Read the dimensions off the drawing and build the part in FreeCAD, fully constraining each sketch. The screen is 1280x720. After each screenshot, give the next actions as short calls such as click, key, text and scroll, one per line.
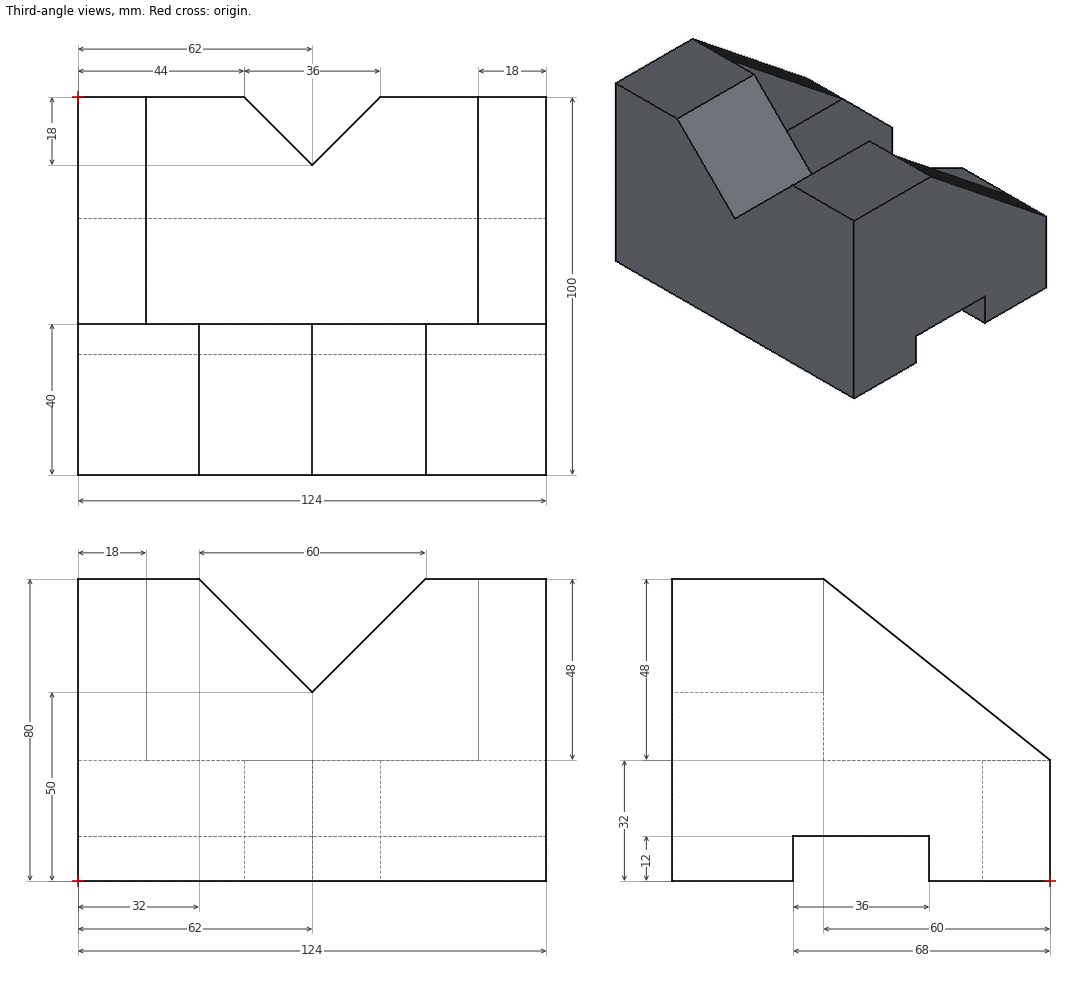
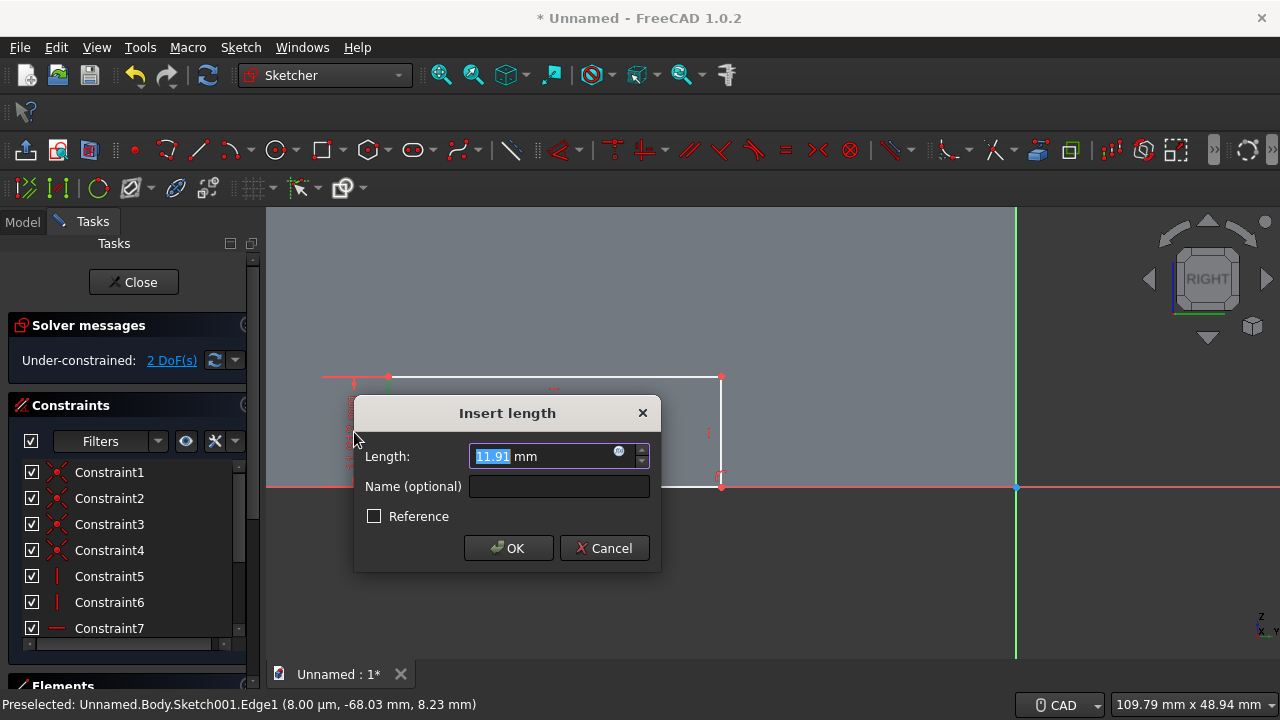
text(12)
key(Return)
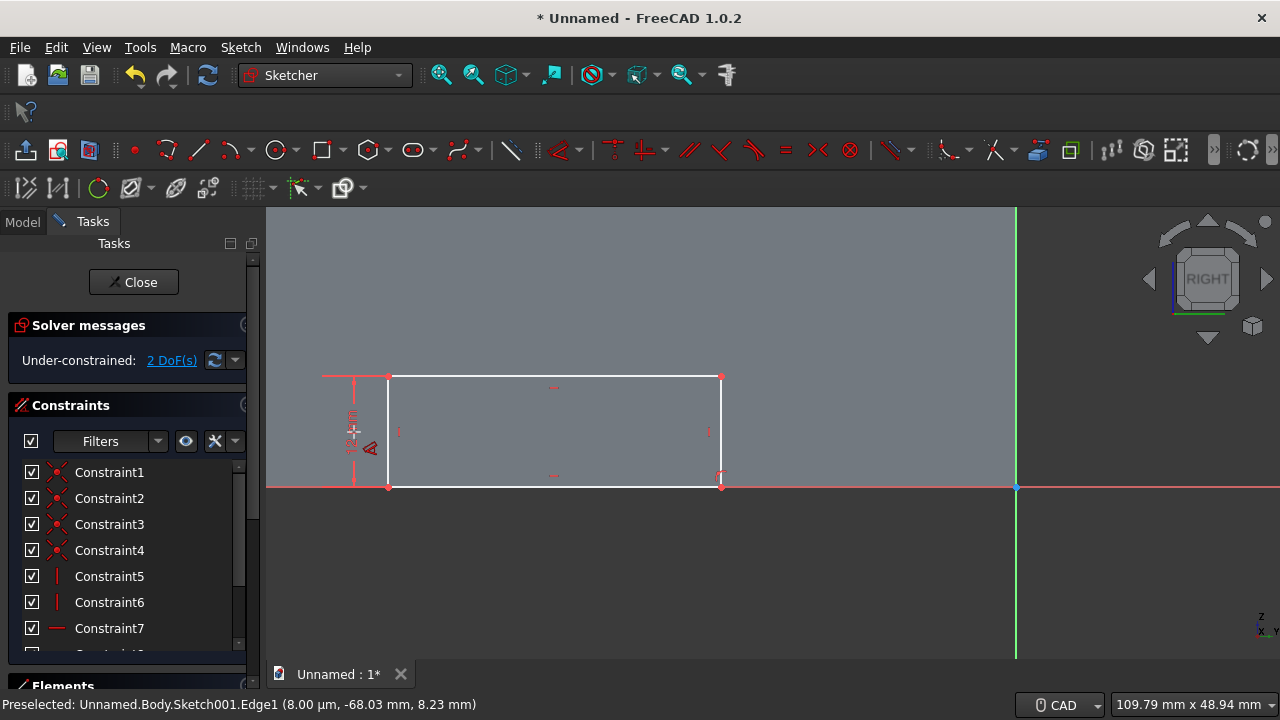
click(488, 487)
click(554, 521)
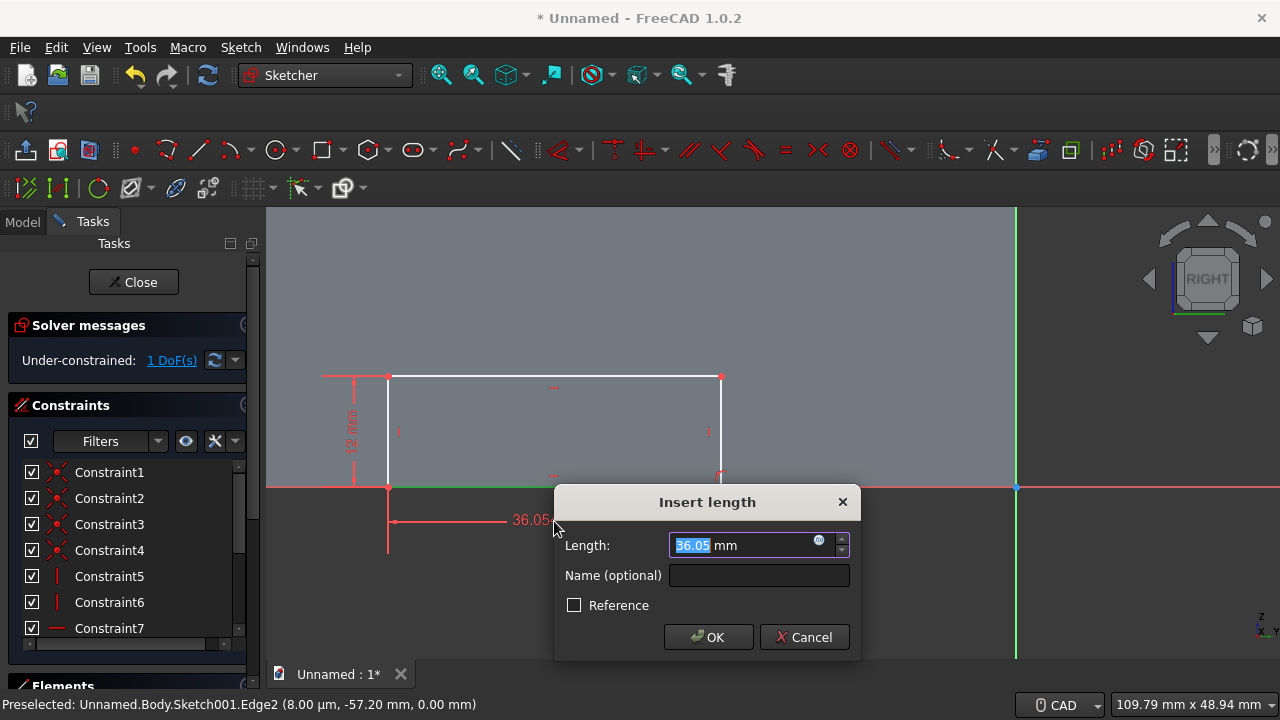
text(36)
key(Return)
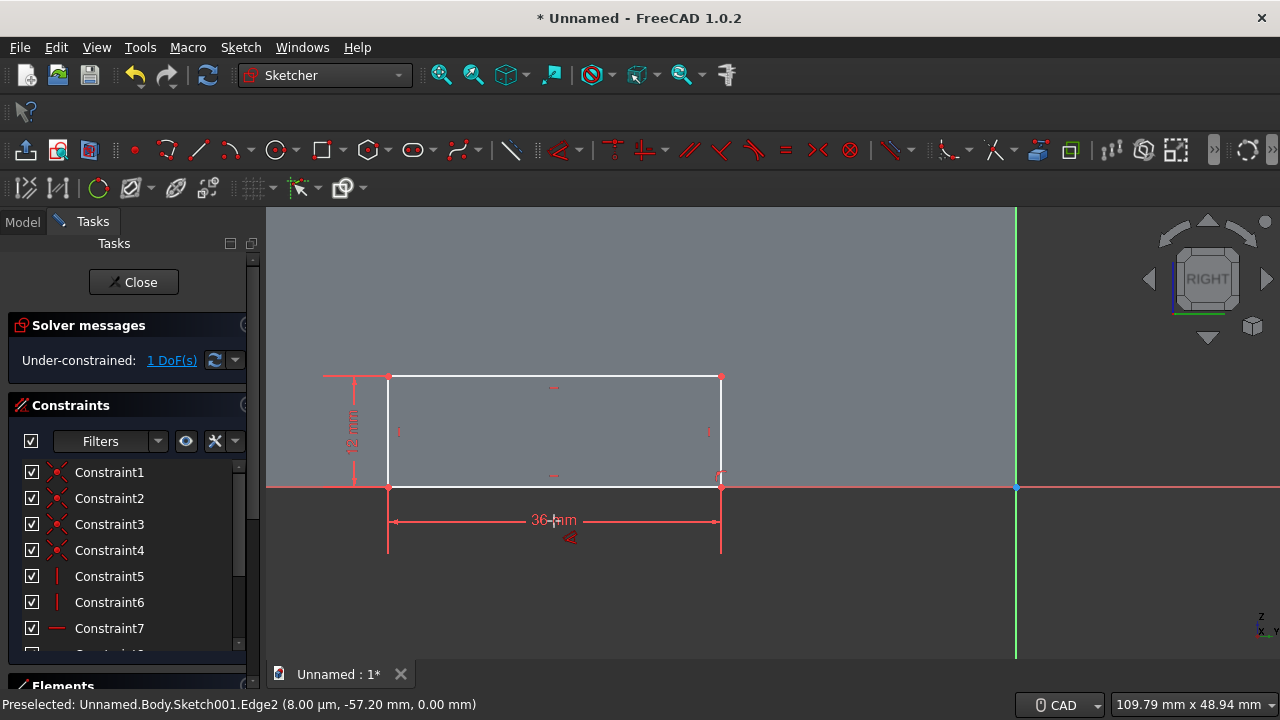
click(388, 376)
click(702, 521)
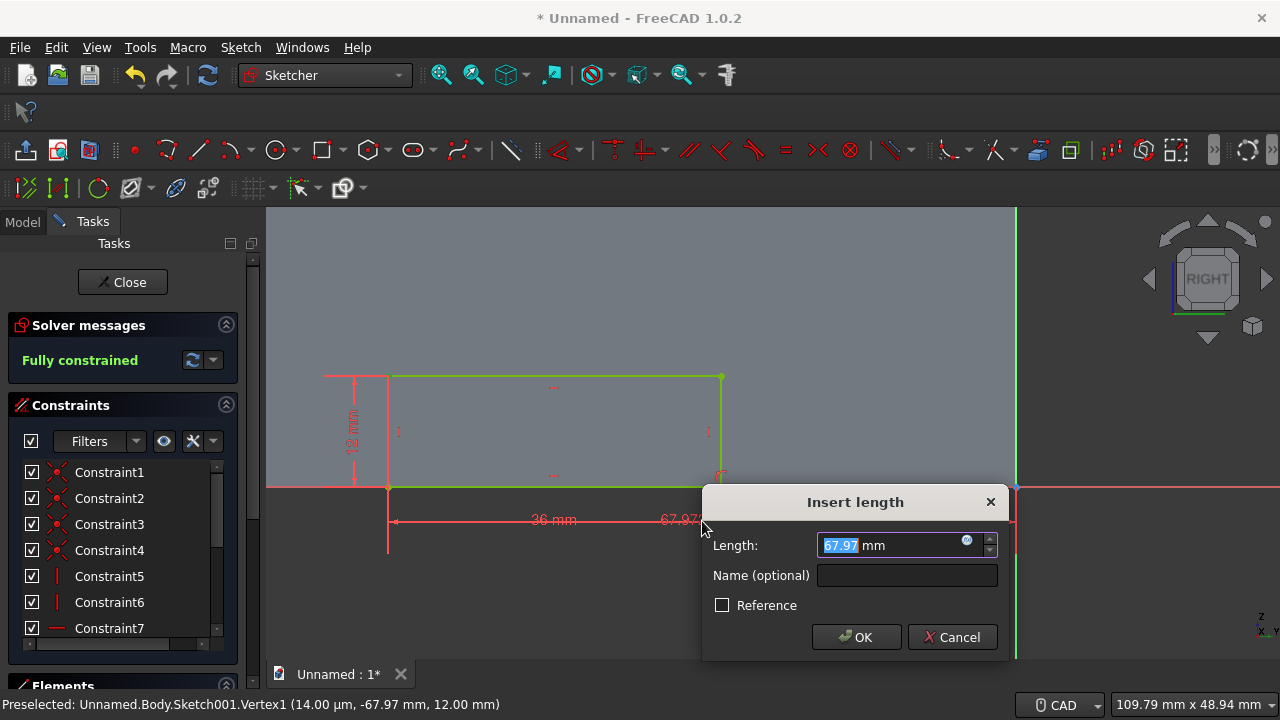
text(68)
key(Return)
key(Escape)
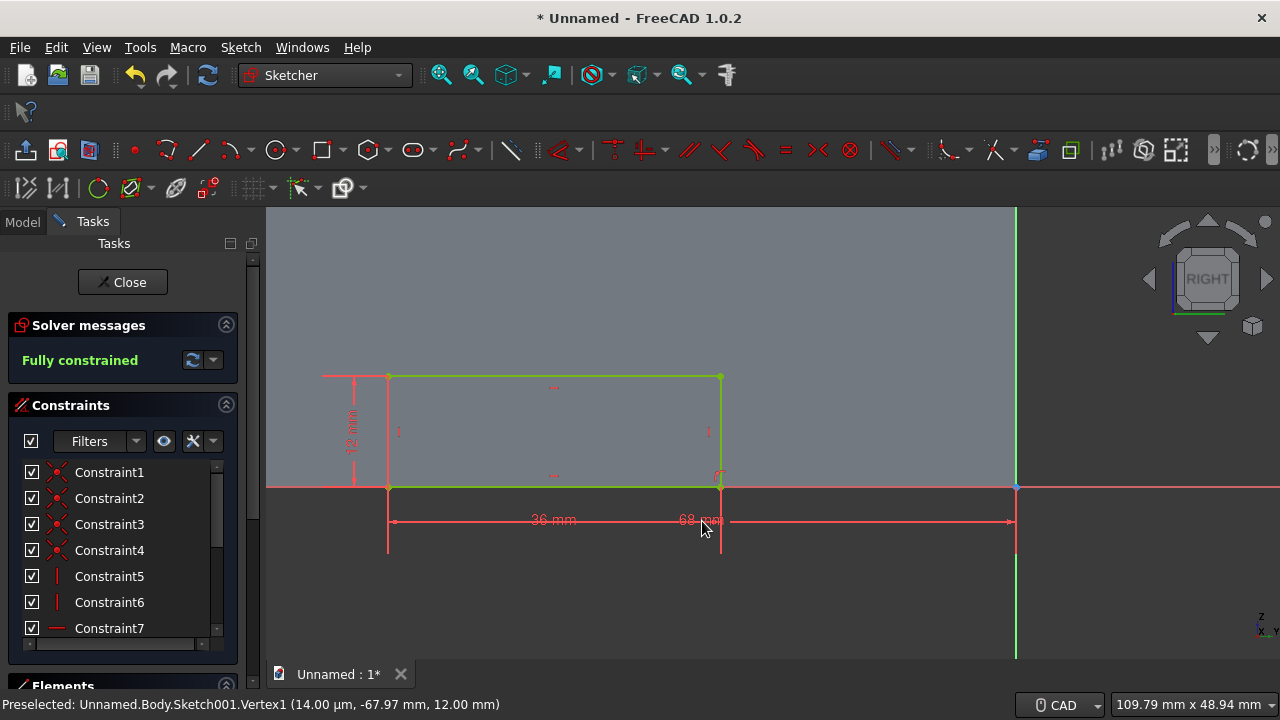
click(123, 282)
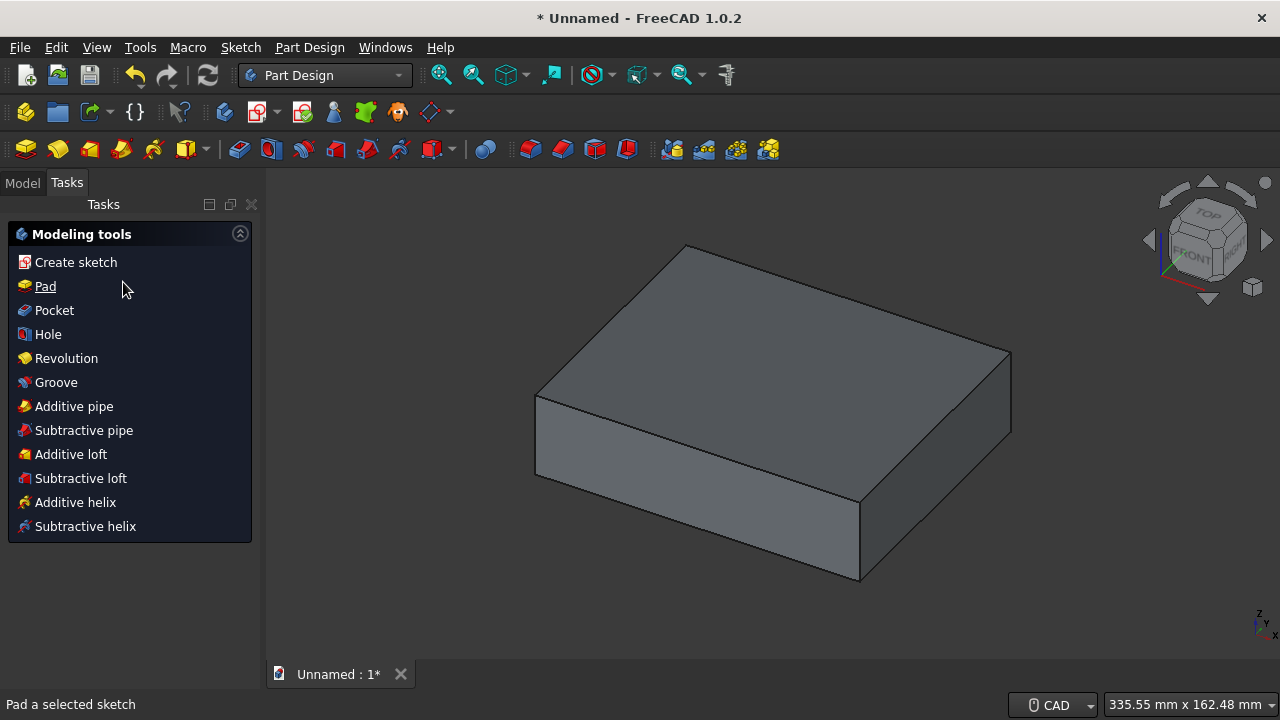
click(240, 150)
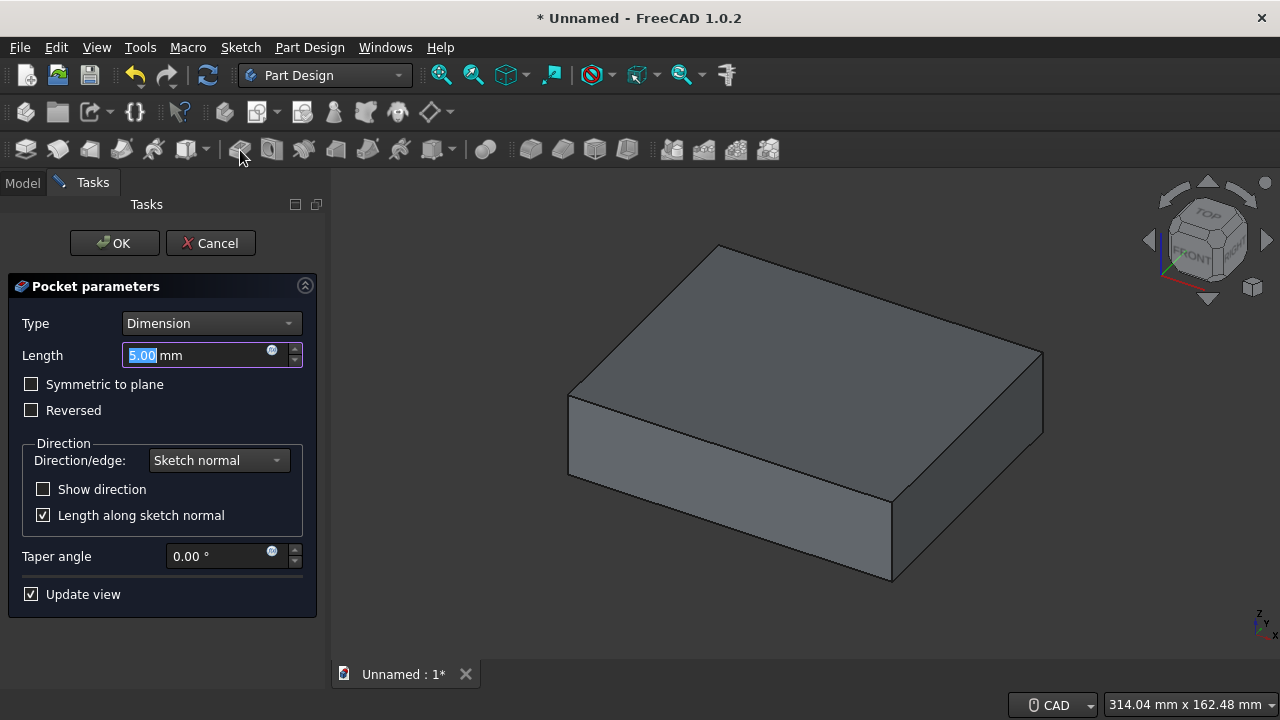
text(124)
key(Tab)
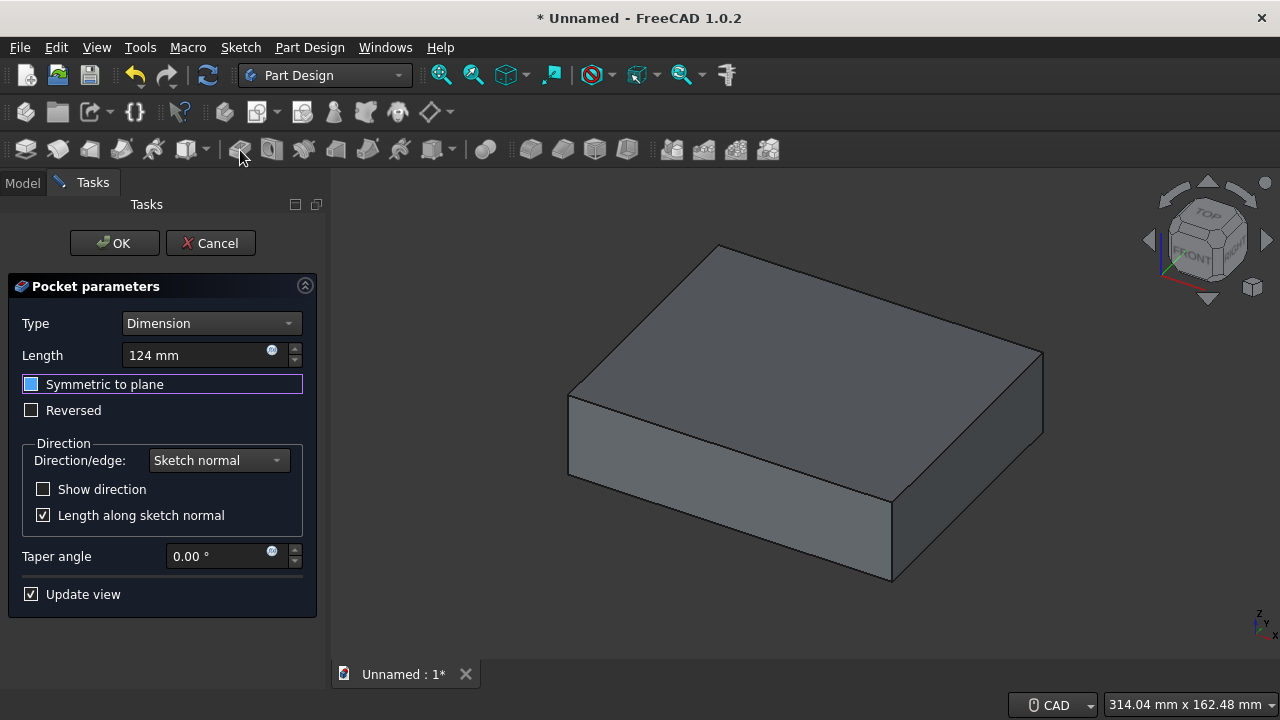
click(30, 410)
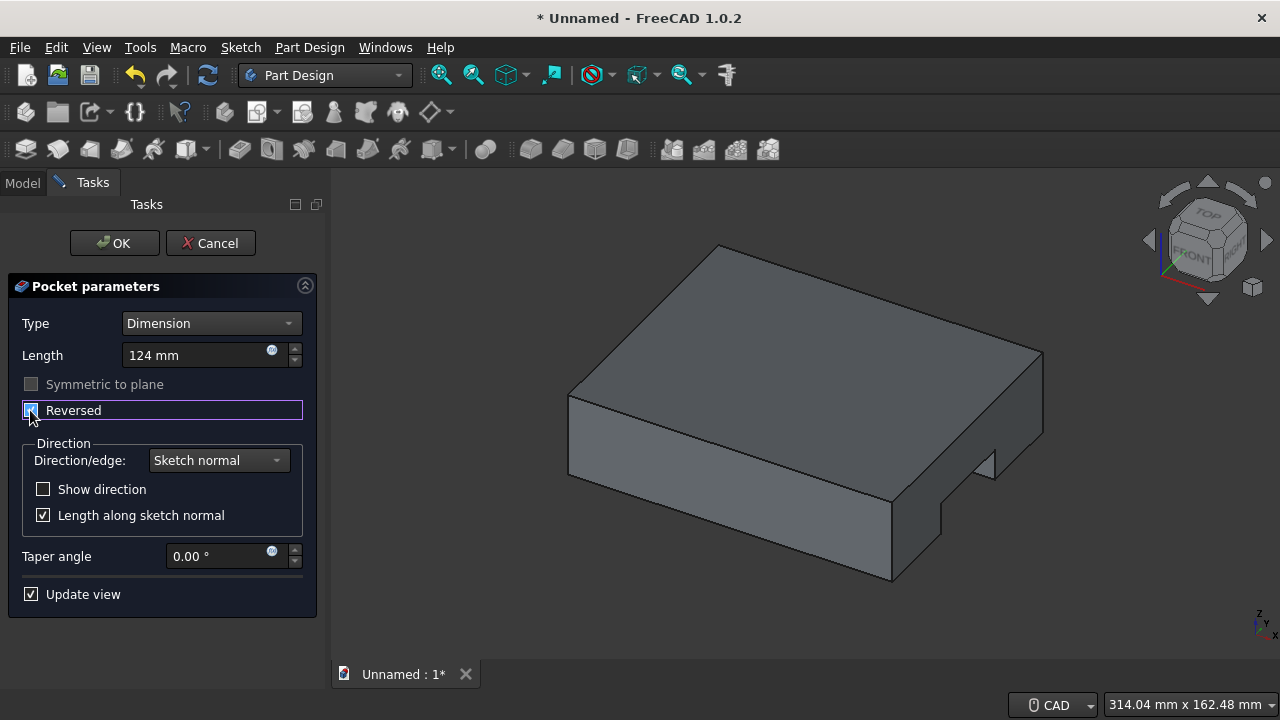
click(115, 243)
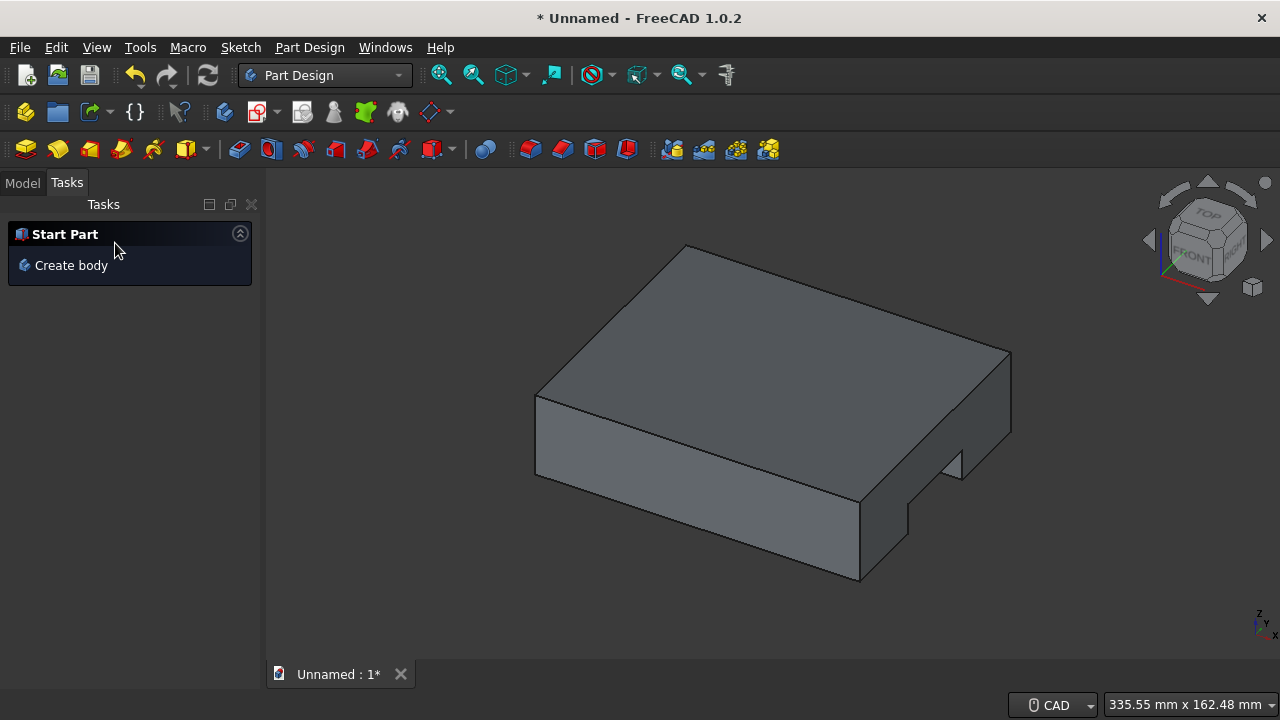
click(790, 518)